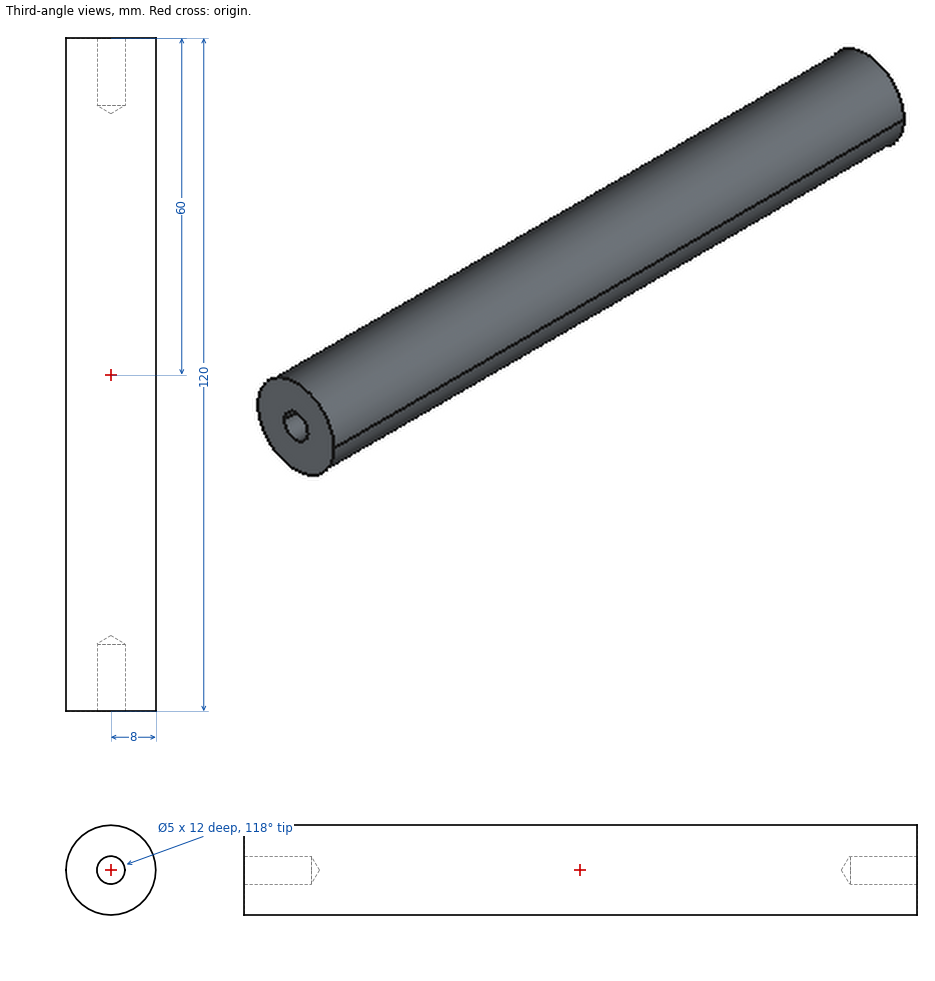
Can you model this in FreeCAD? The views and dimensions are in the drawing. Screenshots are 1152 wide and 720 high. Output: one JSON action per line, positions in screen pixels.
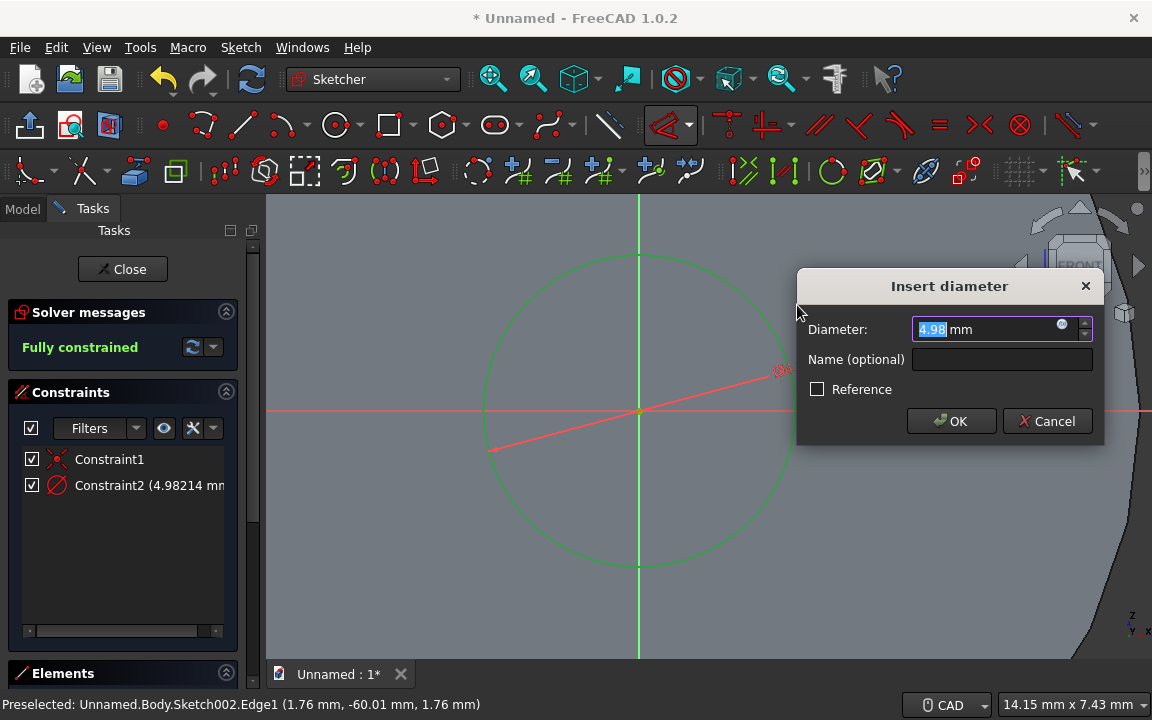
{"action": "type", "text": "5"}
{"action": "key", "text": "Return"}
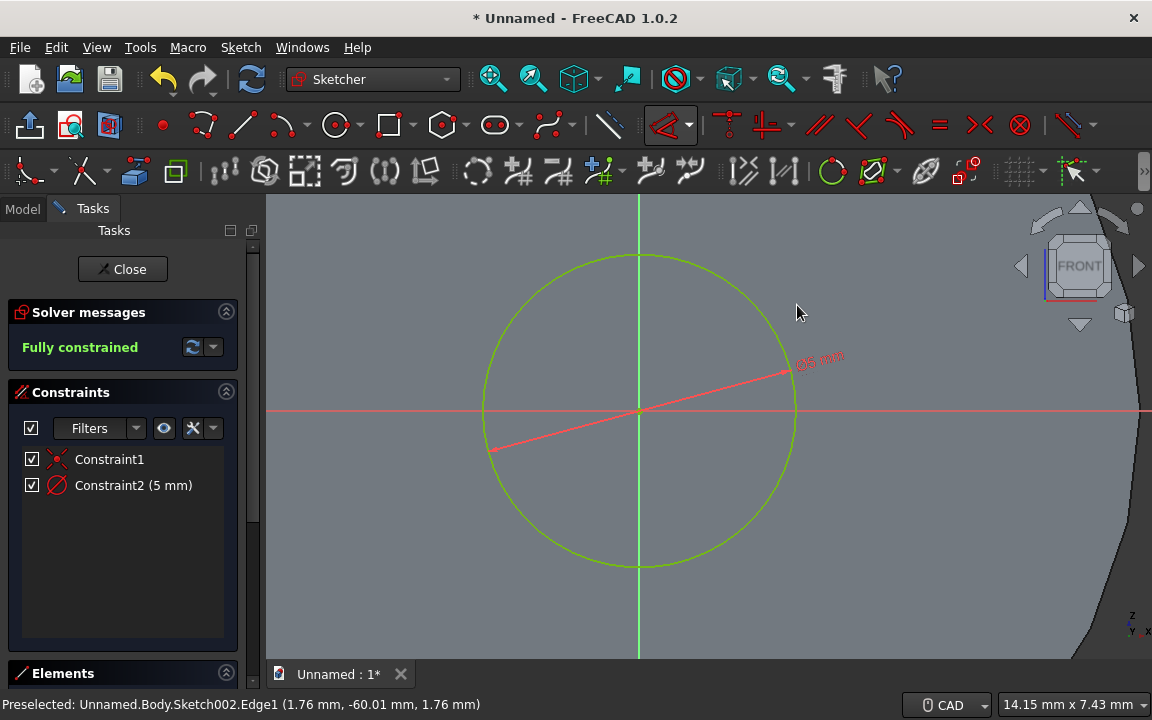
{"action": "left_click", "coordinate": [123, 269]}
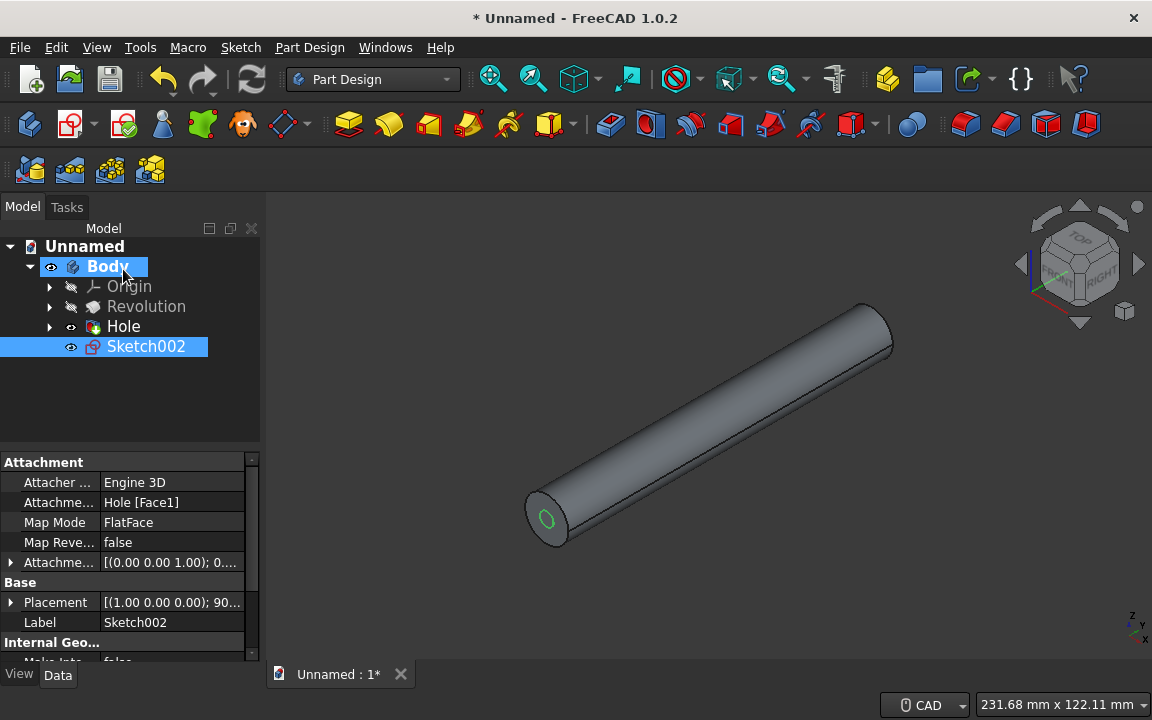
{"action": "left_click", "coordinate": [652, 124]}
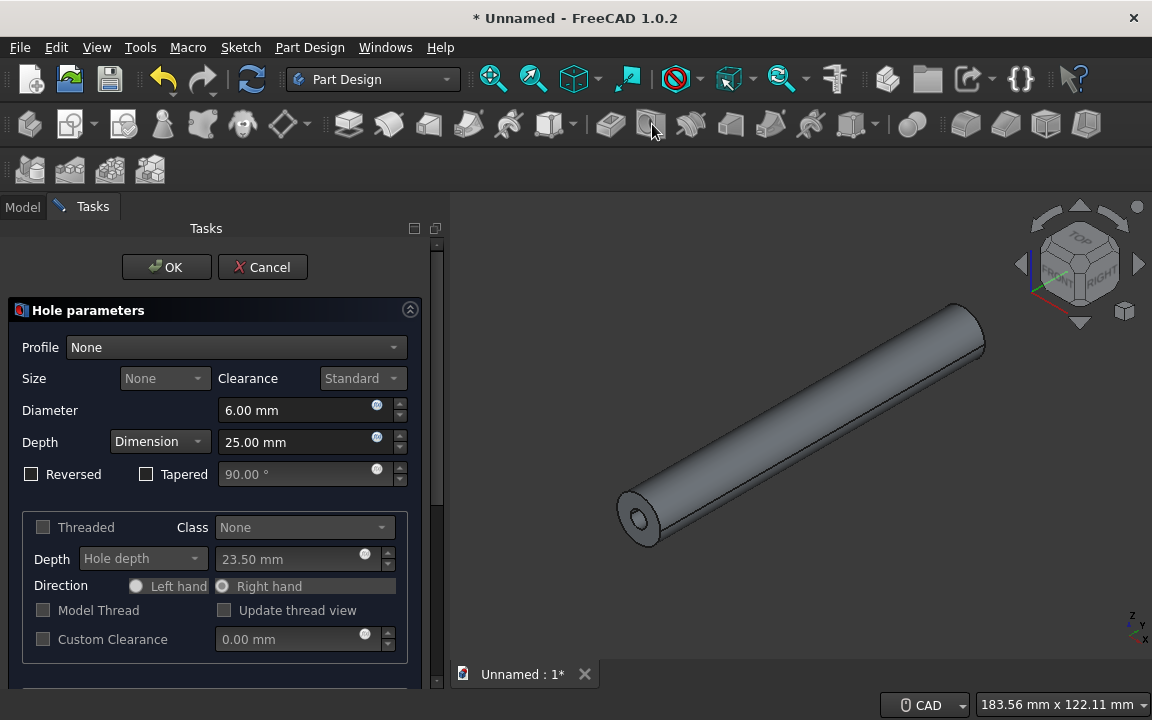
{"action": "triple_click", "coordinate": [305, 410]}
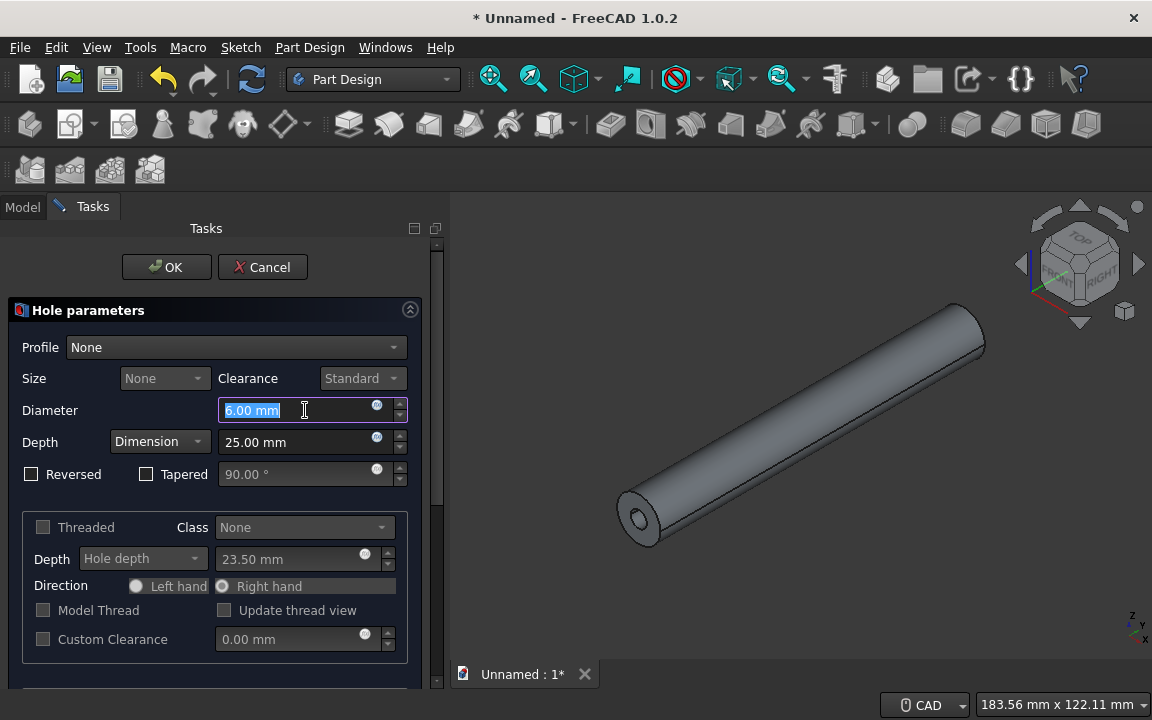
{"action": "type", "text": "5"}
{"action": "key", "text": "Tab"}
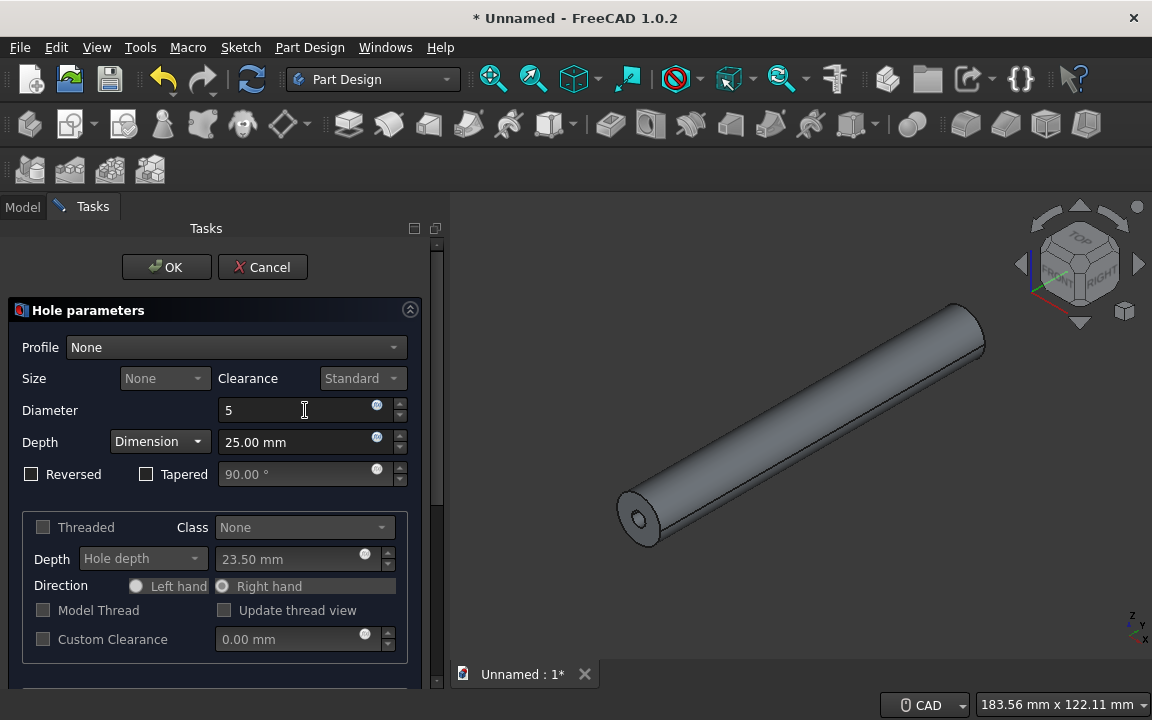
{"action": "triple_click", "coordinate": [305, 442]}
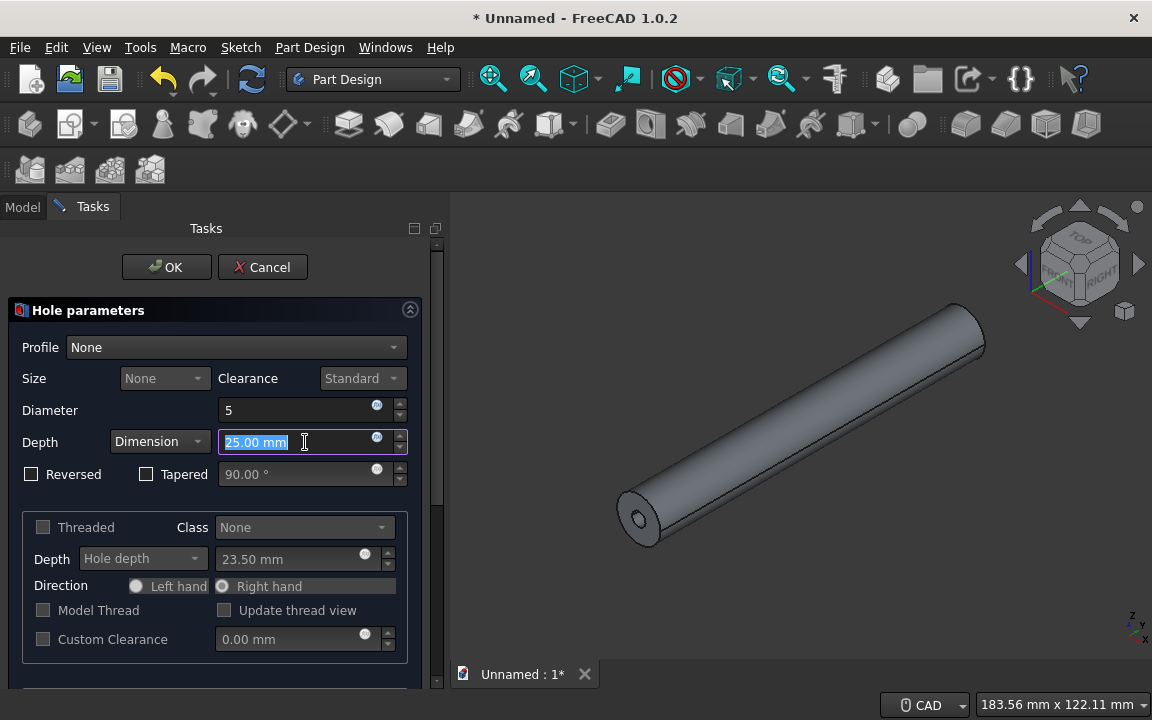
{"action": "type", "text": "12"}
{"action": "key", "text": "Tab"}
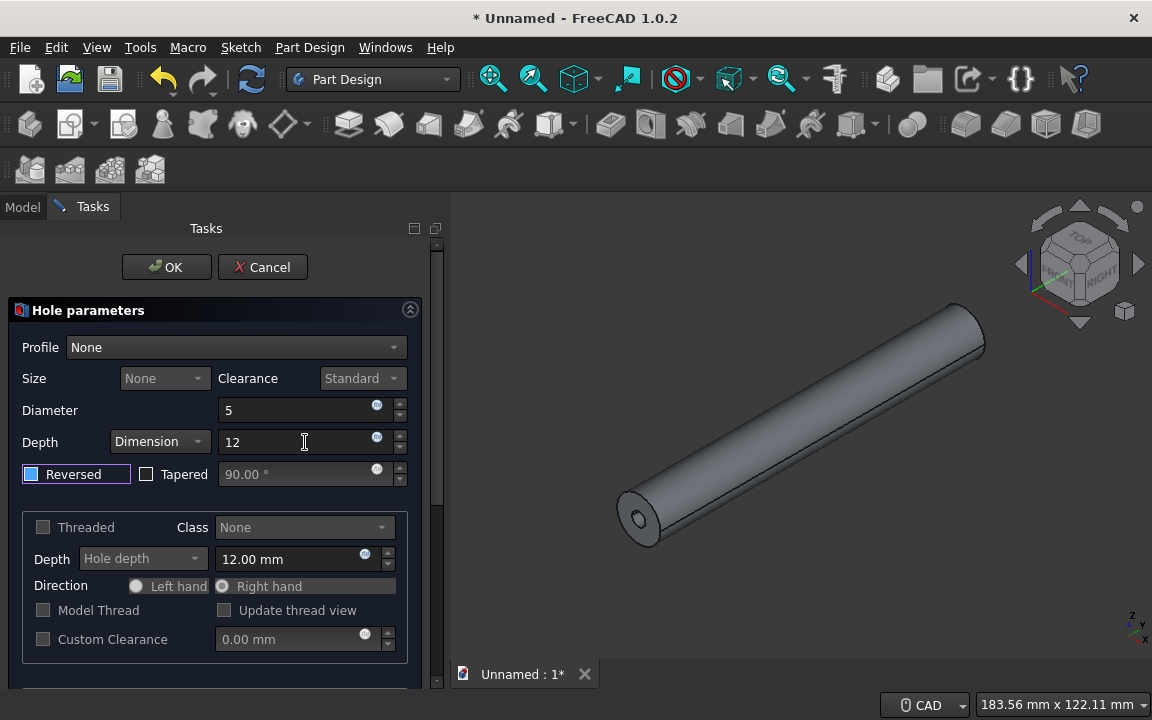
{"action": "left_click", "coordinate": [167, 267]}